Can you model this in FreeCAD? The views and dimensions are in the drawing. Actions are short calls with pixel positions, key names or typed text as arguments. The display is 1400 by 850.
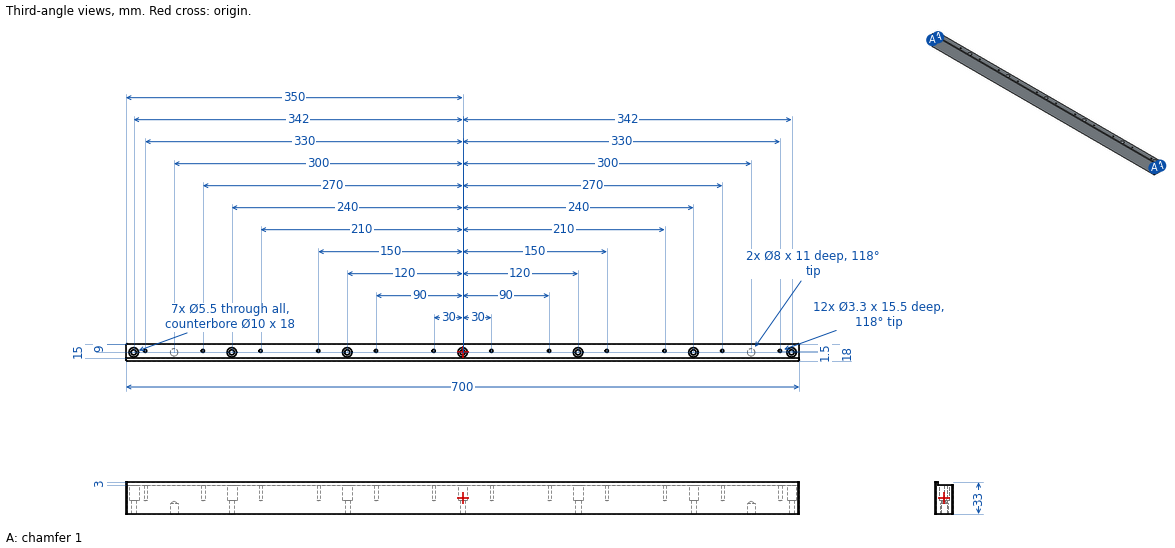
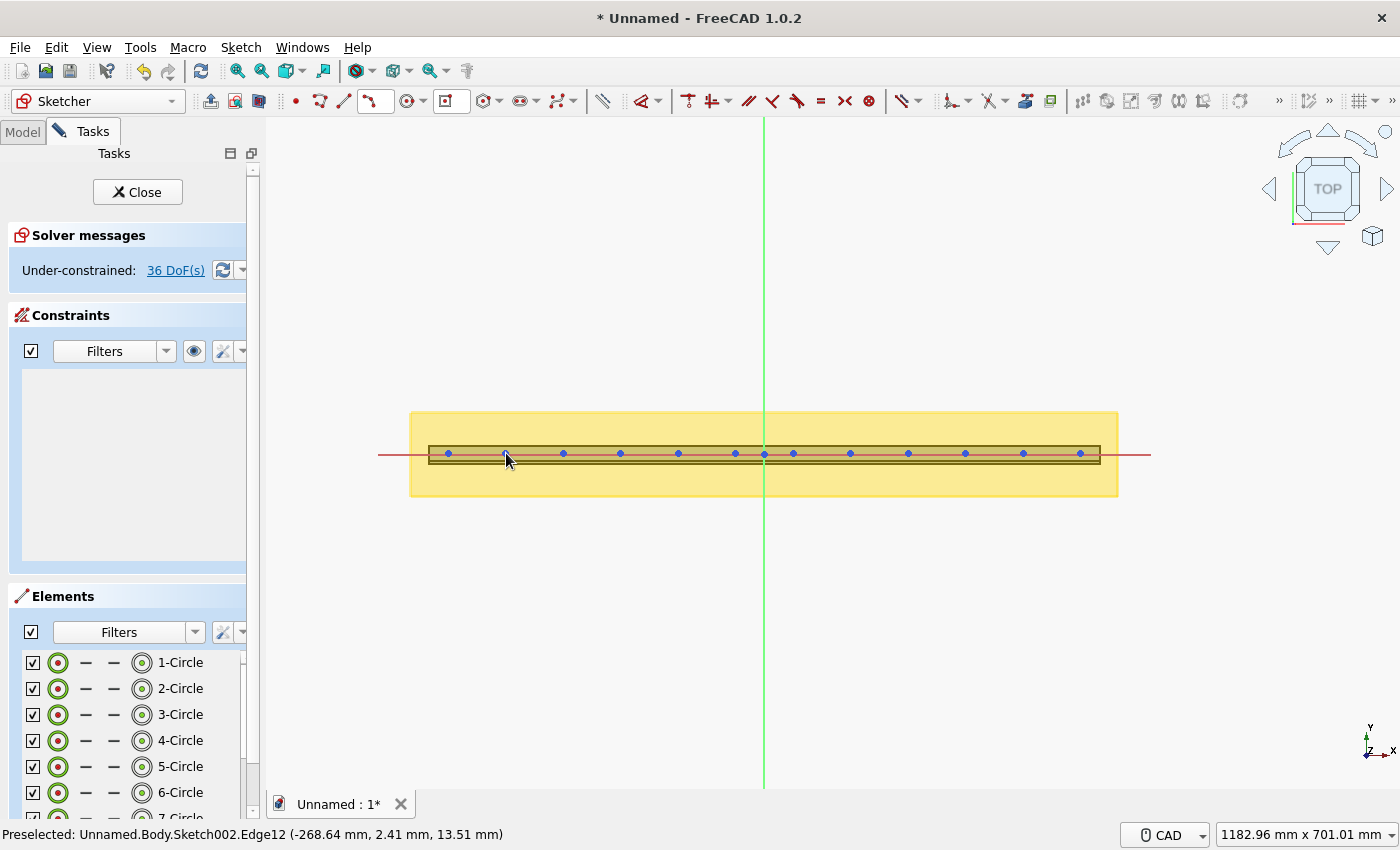
scroll(1082, 452, up, 11)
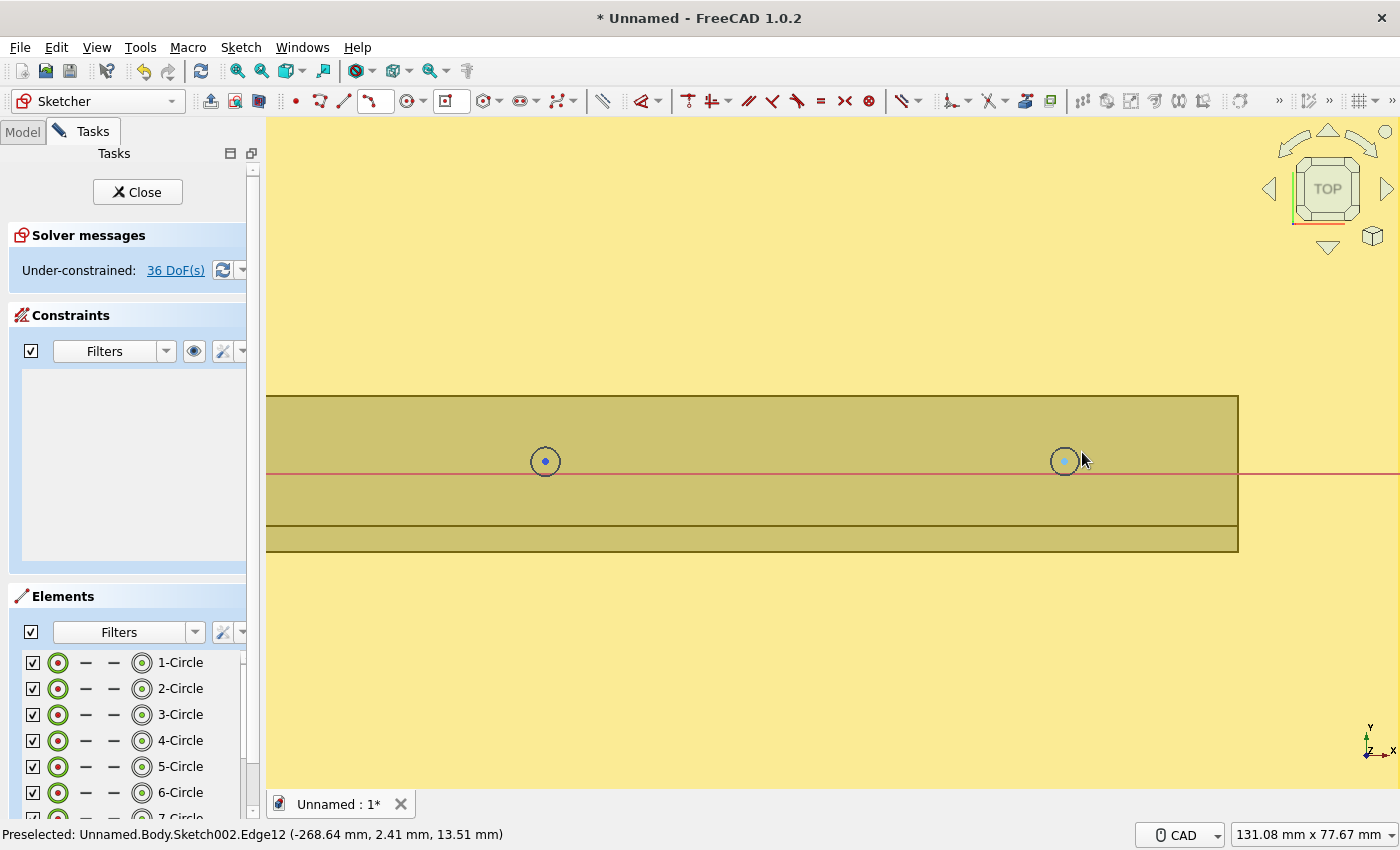
click(1075, 452)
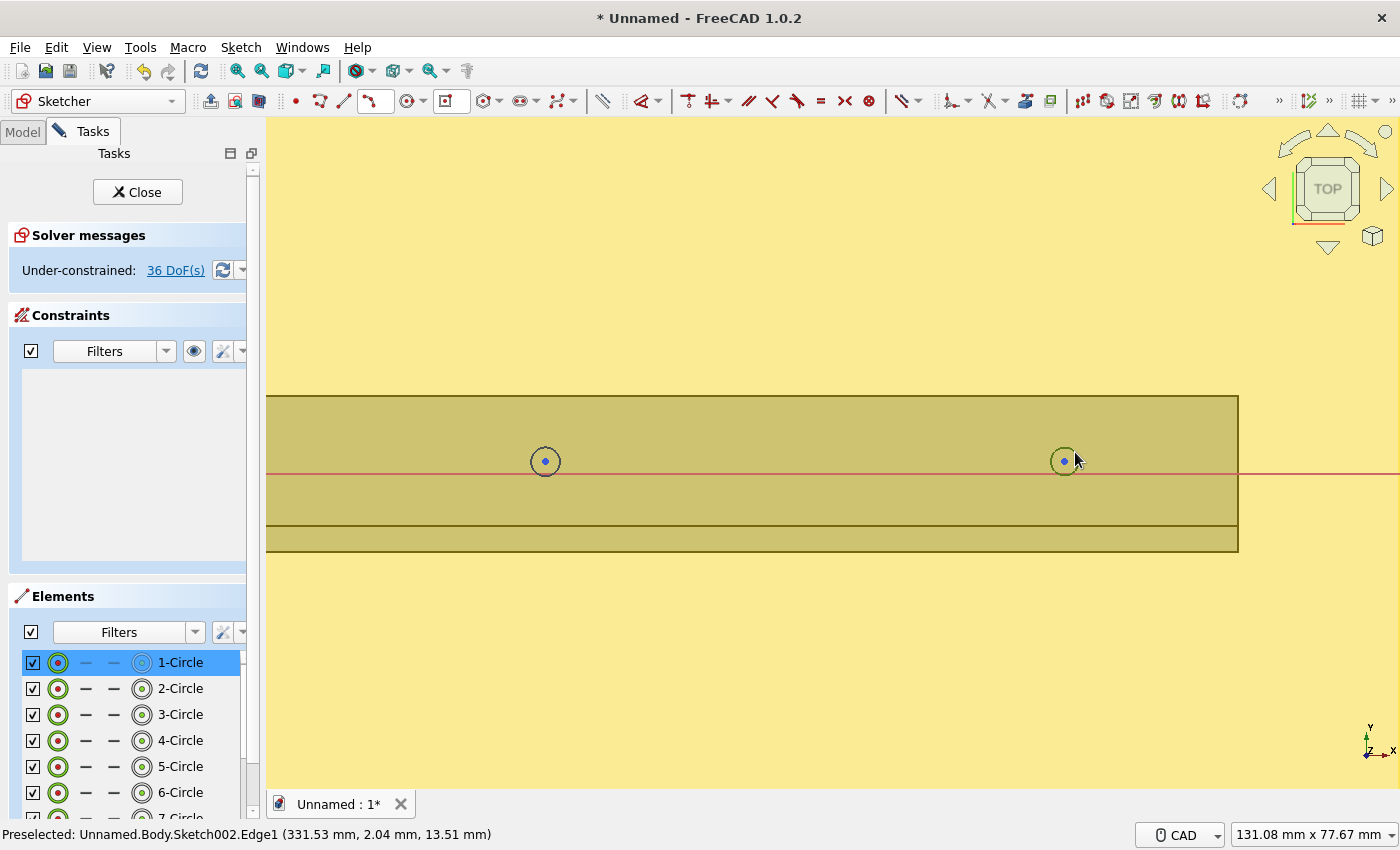
click(556, 452)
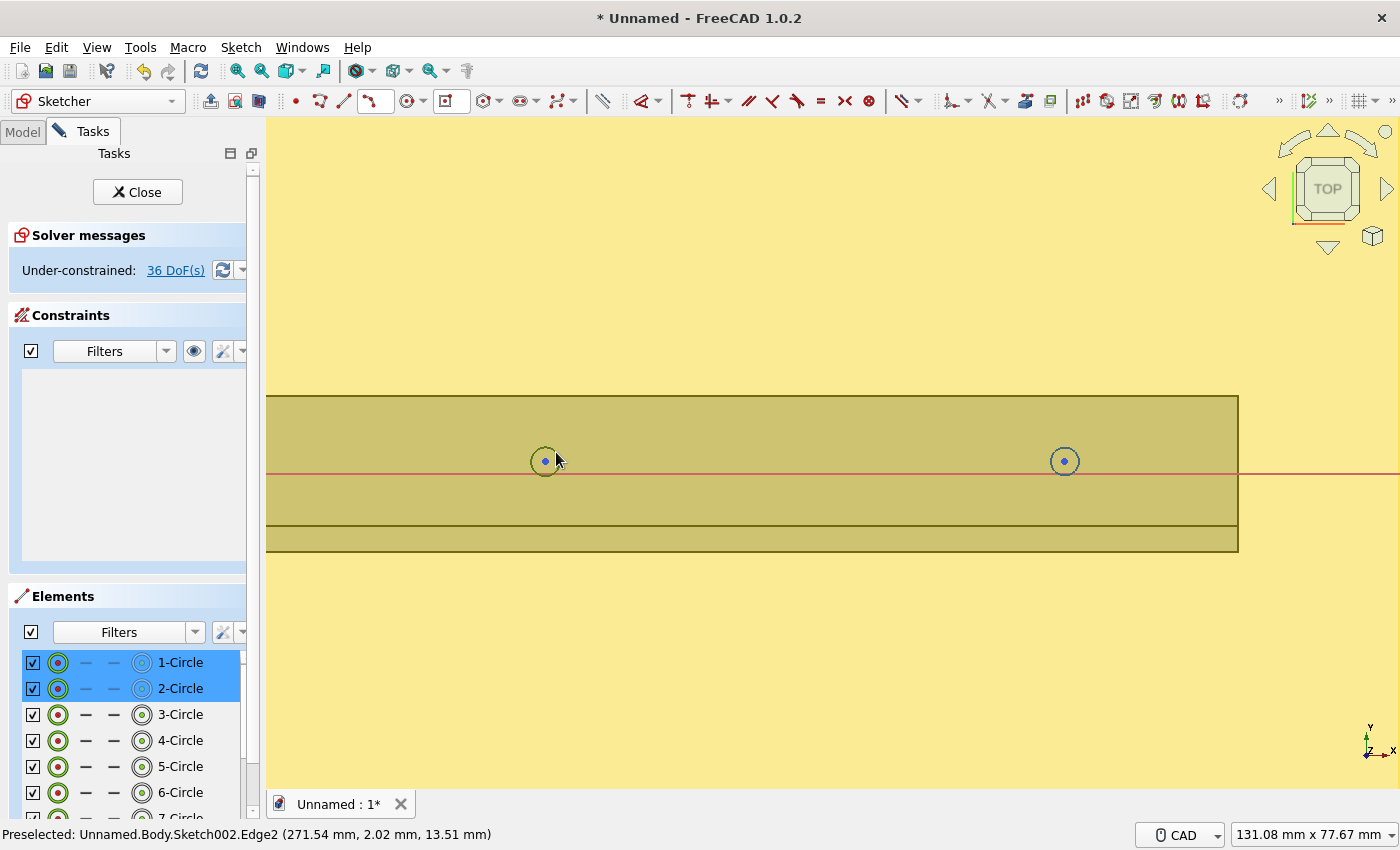
scroll(1083, 452, down, 11)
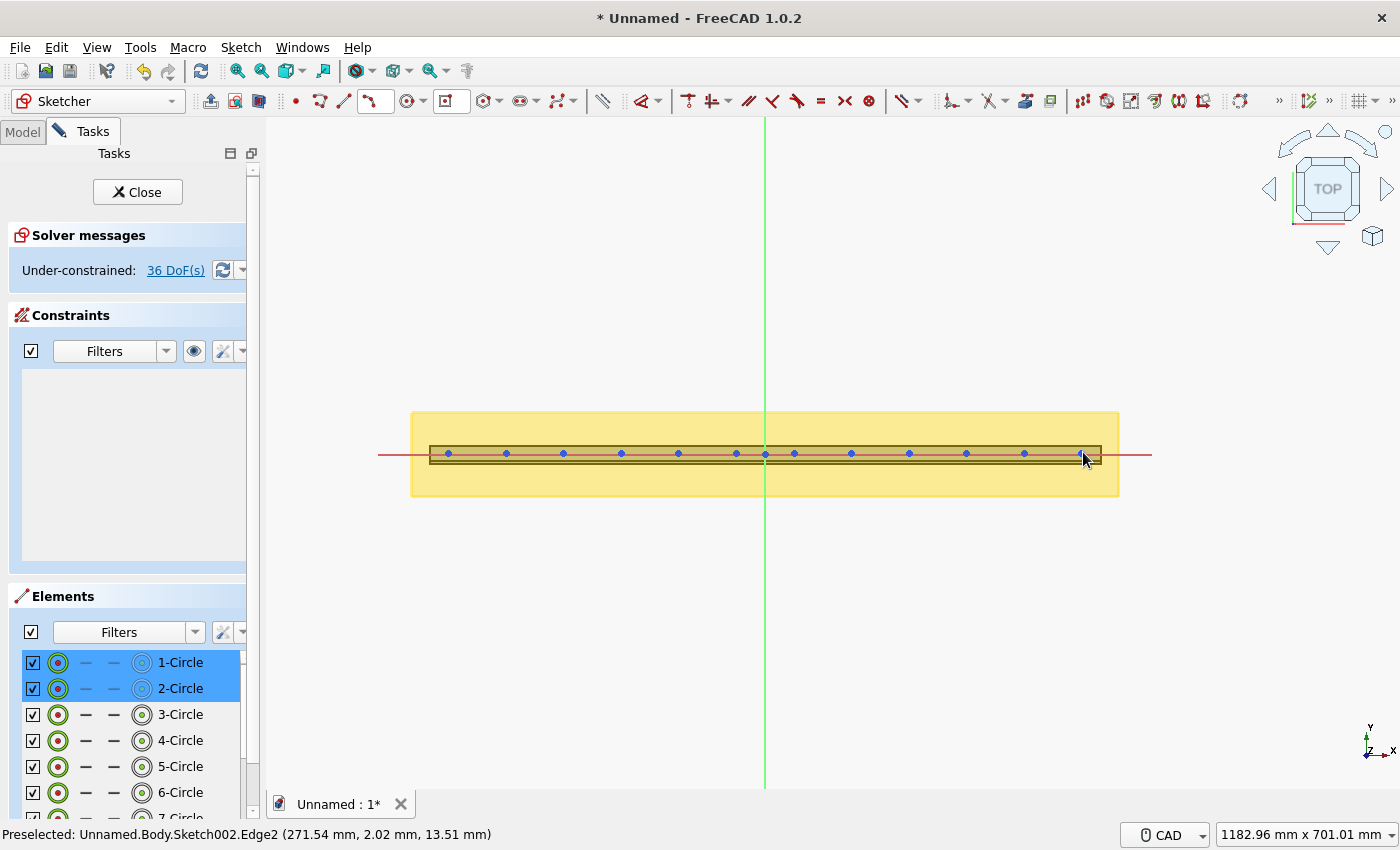
scroll(968, 452, up, 11)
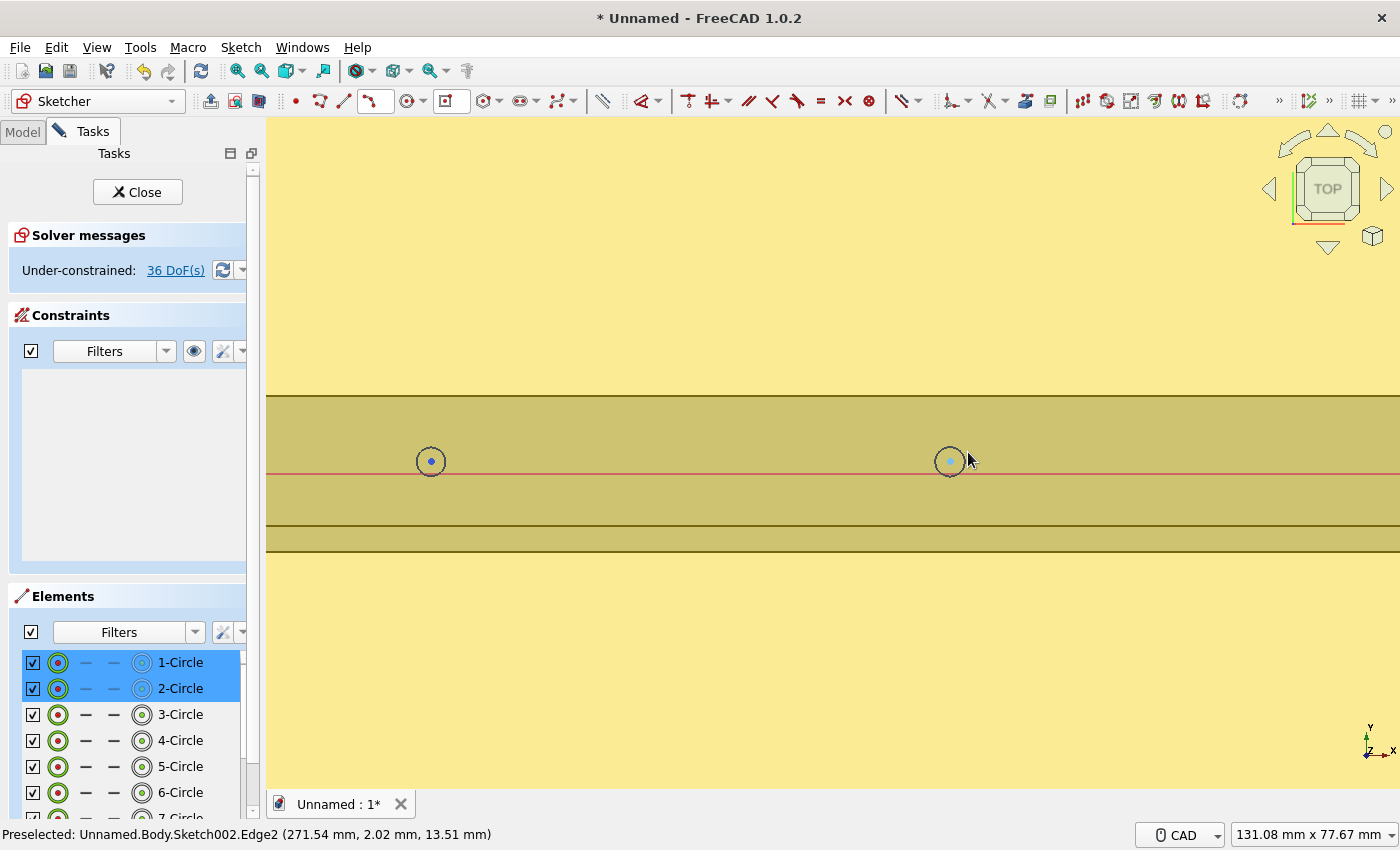
click(960, 451)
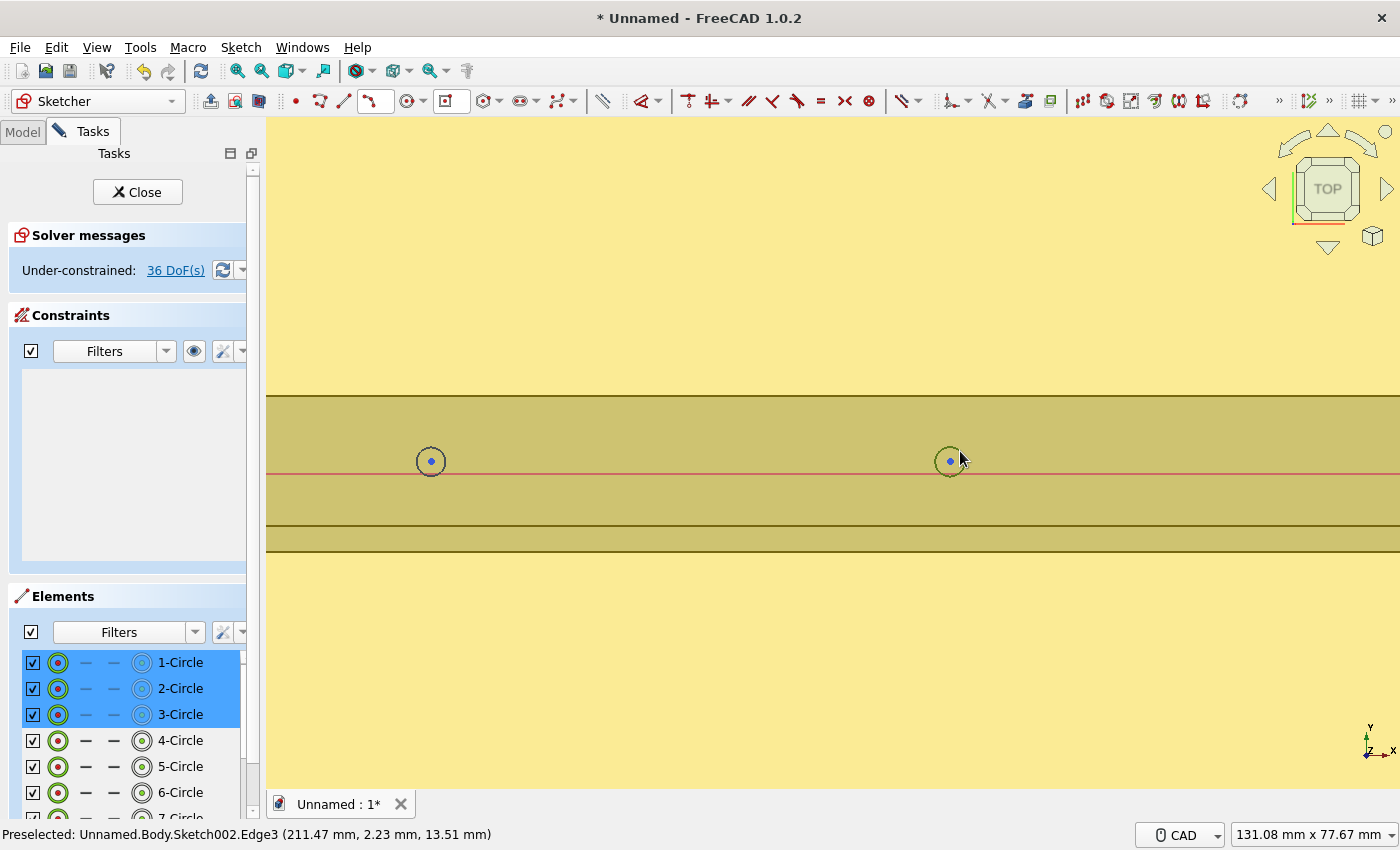
click(441, 452)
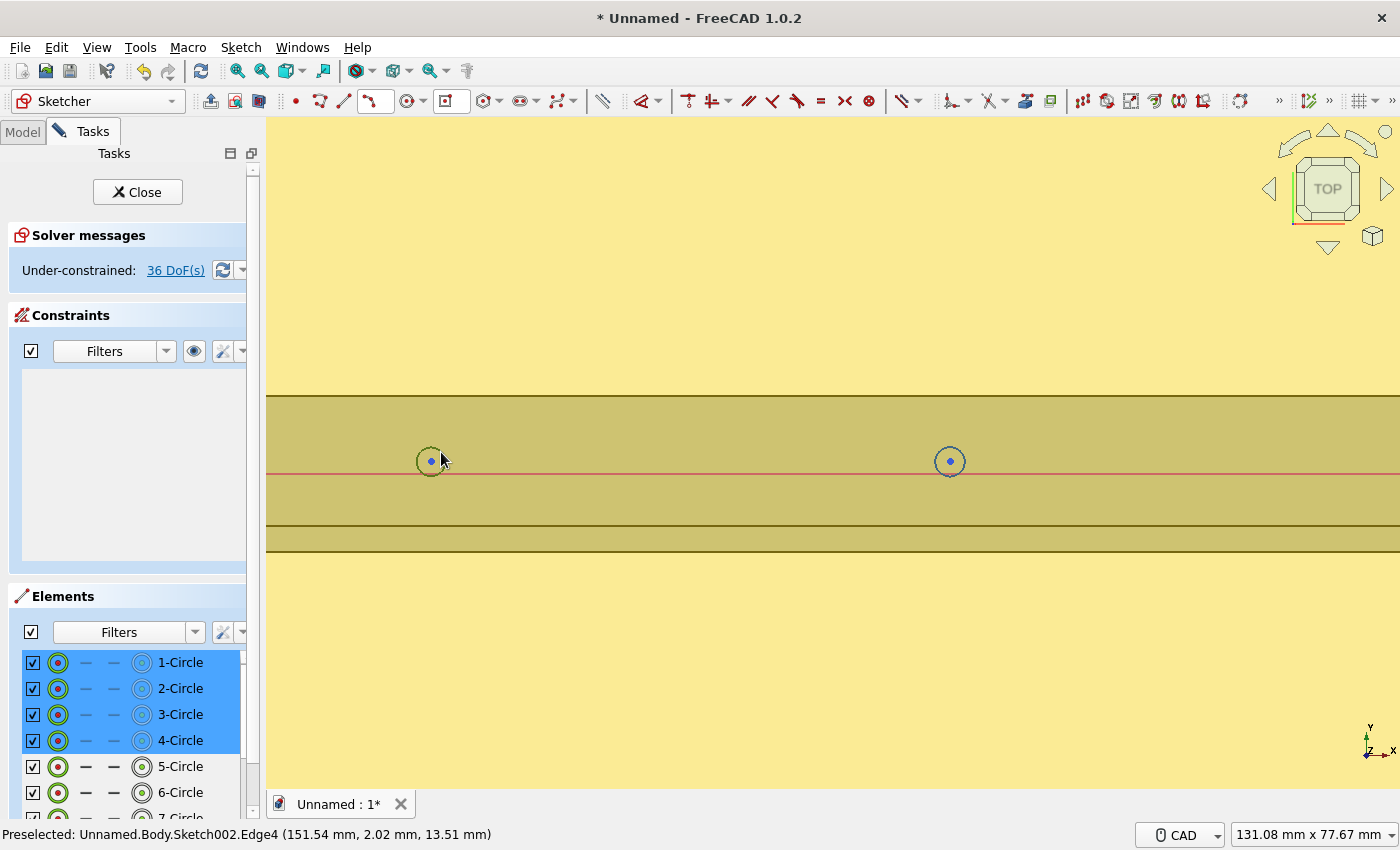
scroll(968, 452, down, 11)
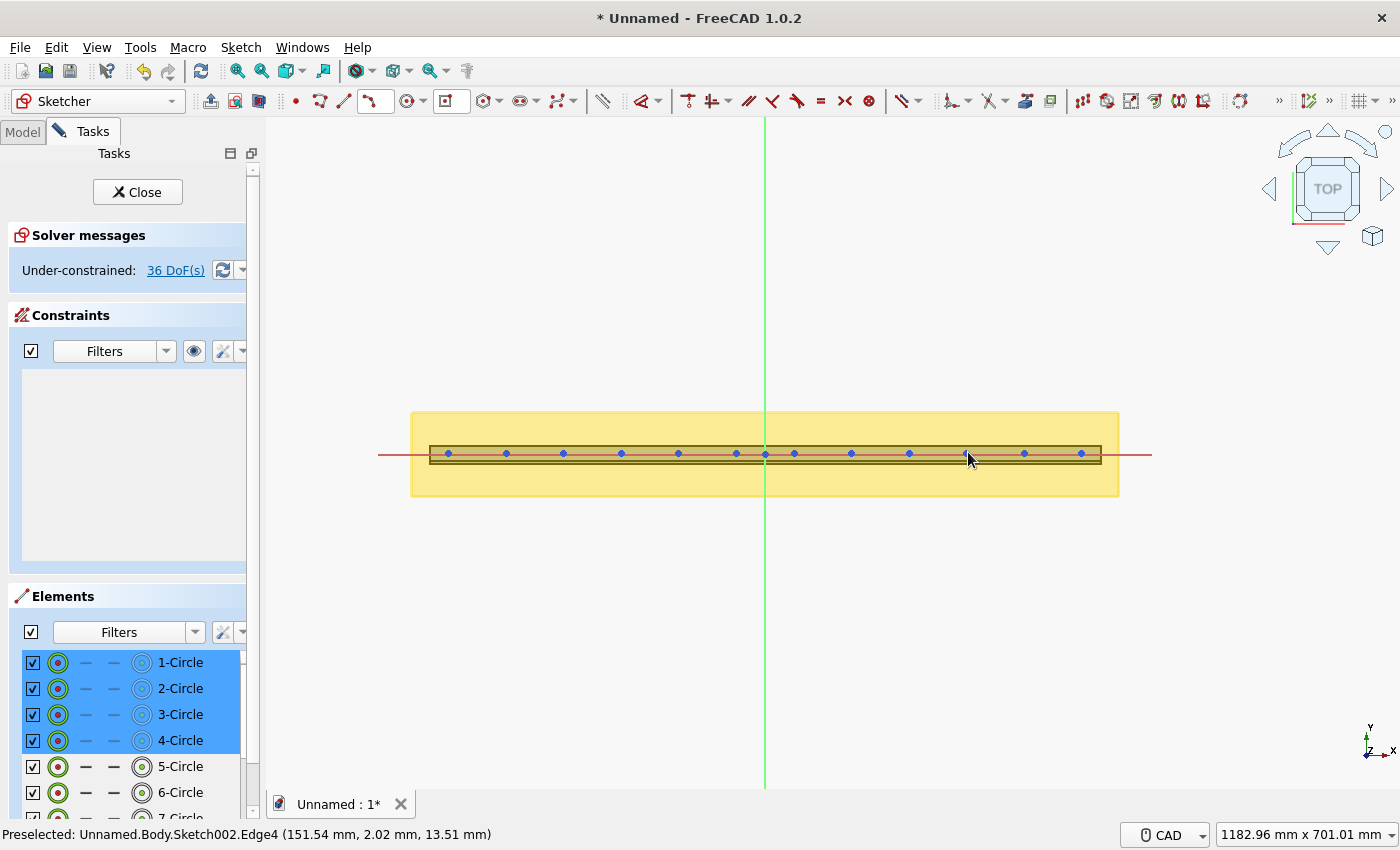
scroll(853, 452, up, 11)